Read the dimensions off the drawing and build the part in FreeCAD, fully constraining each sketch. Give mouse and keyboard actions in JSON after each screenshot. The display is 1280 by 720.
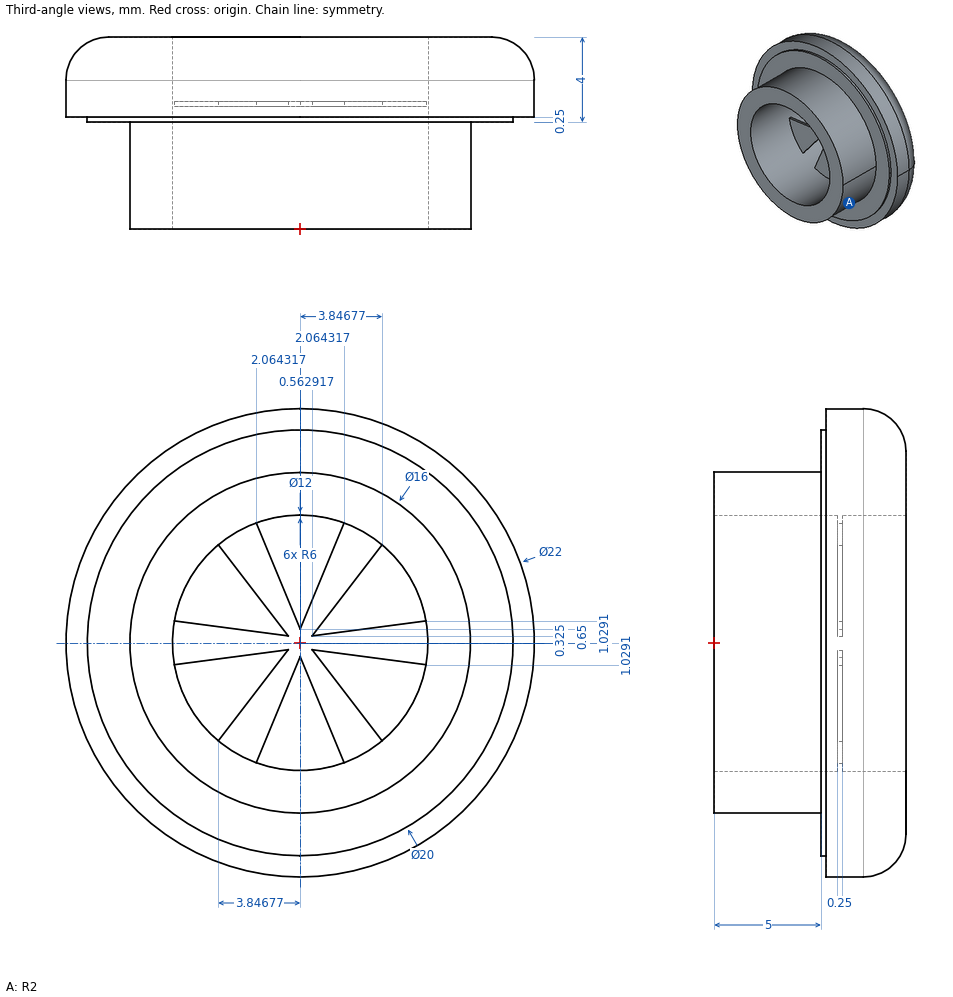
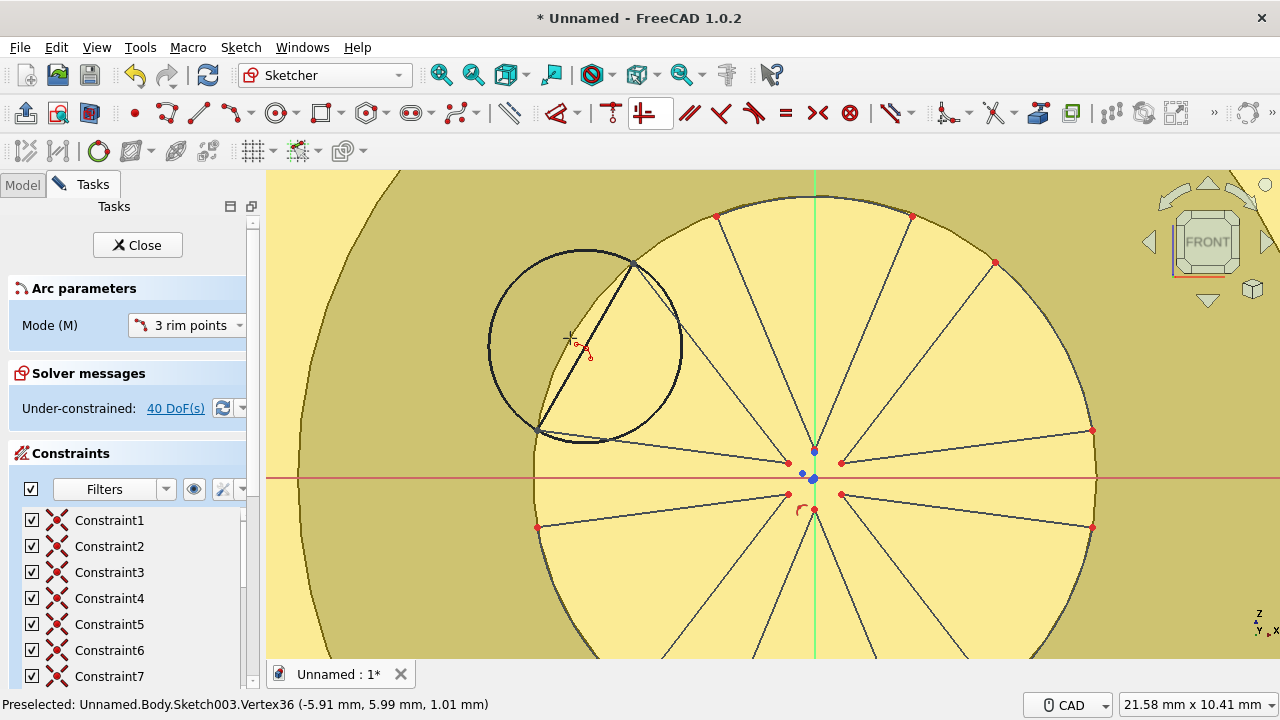
{"action": "left_click", "coordinate": [571, 337]}
{"action": "key", "text": "Escape"}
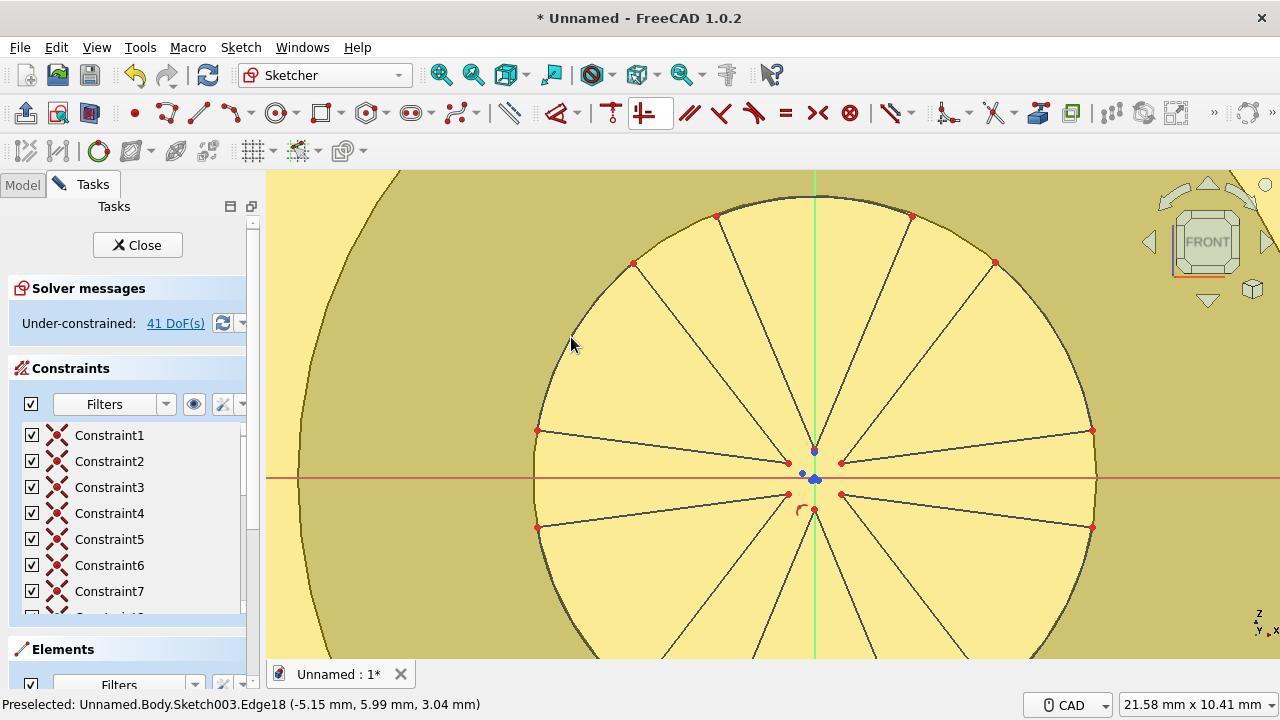
{"action": "left_click", "coordinate": [855, 200]}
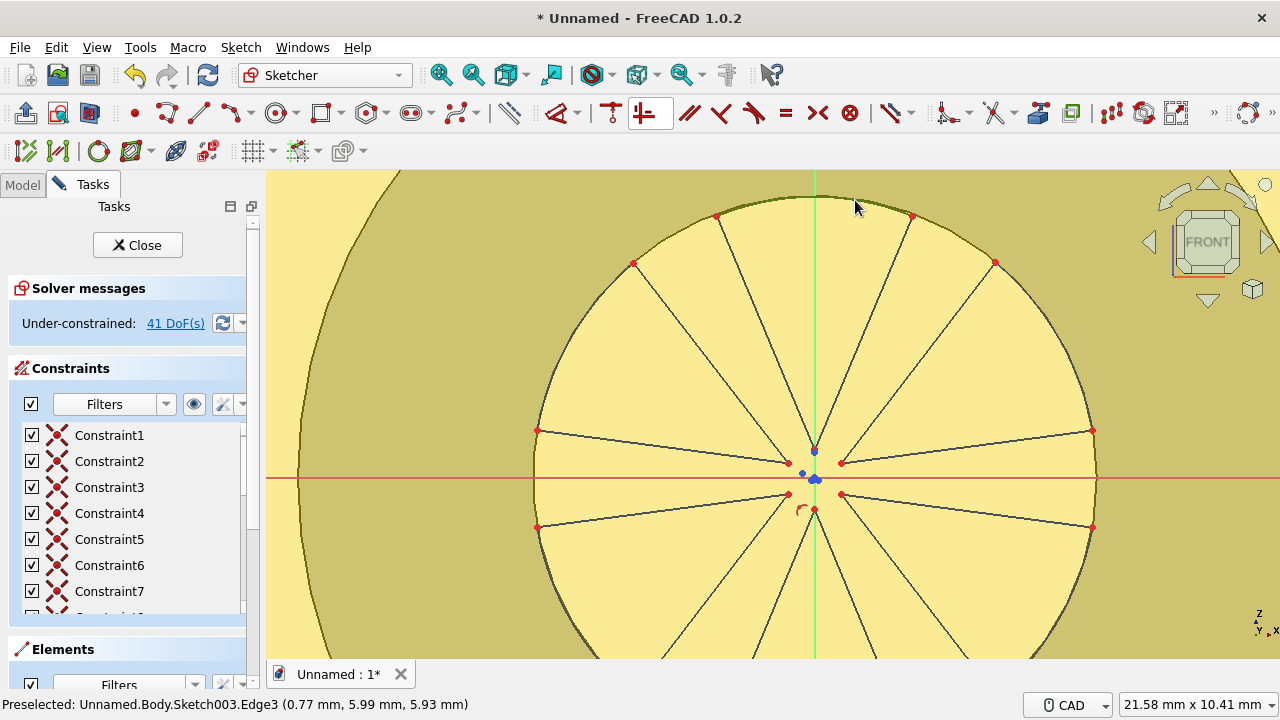
{"action": "left_click", "coordinate": [1076, 374]}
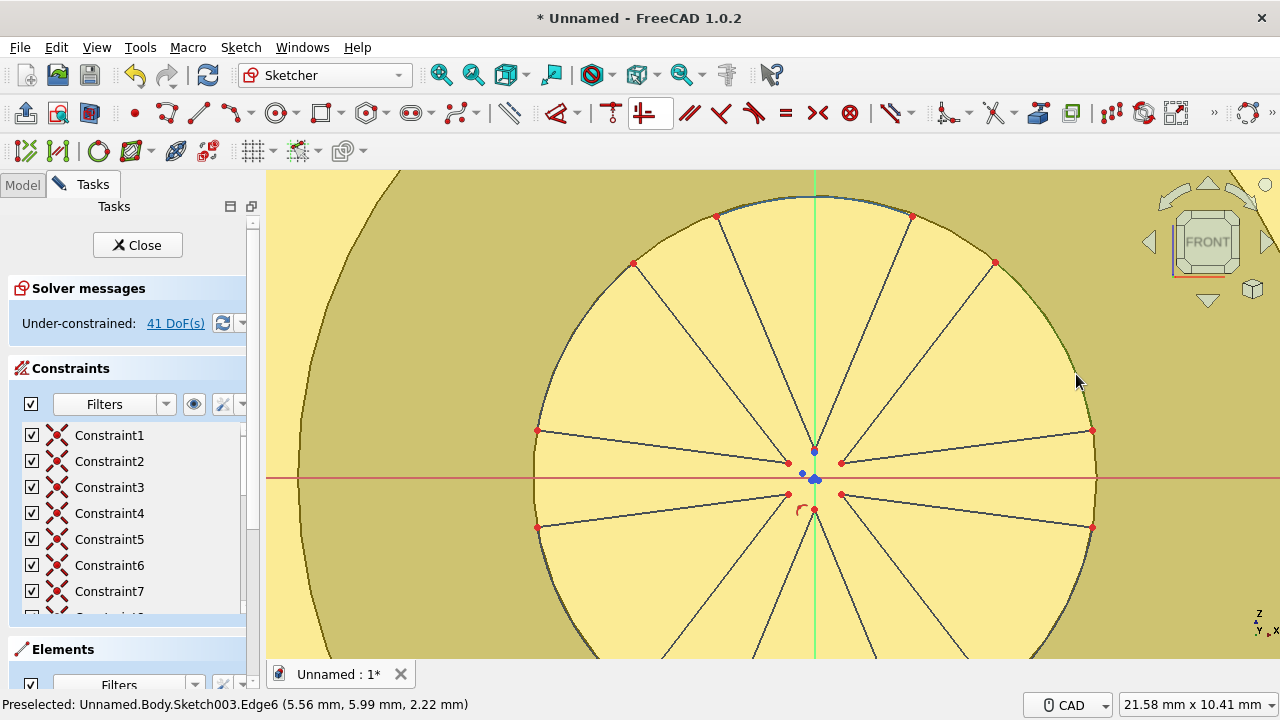
{"action": "key", "text": "c"}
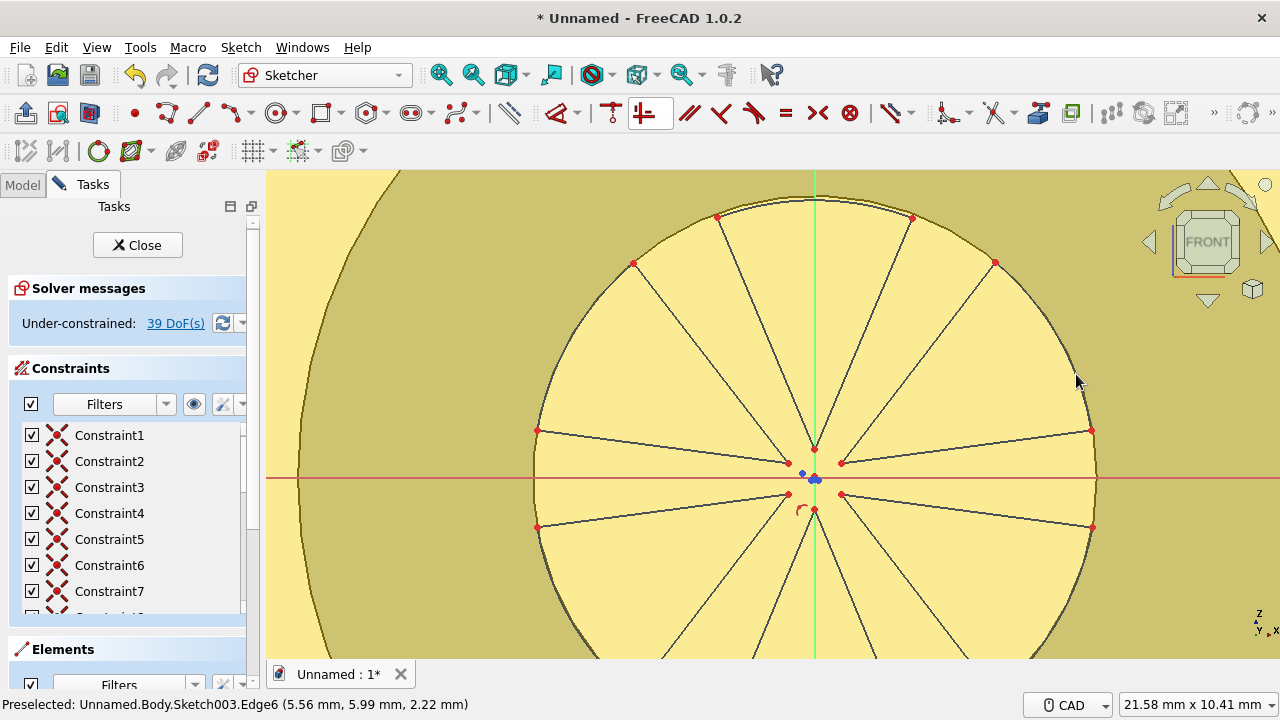
{"action": "left_click", "coordinate": [855, 203]}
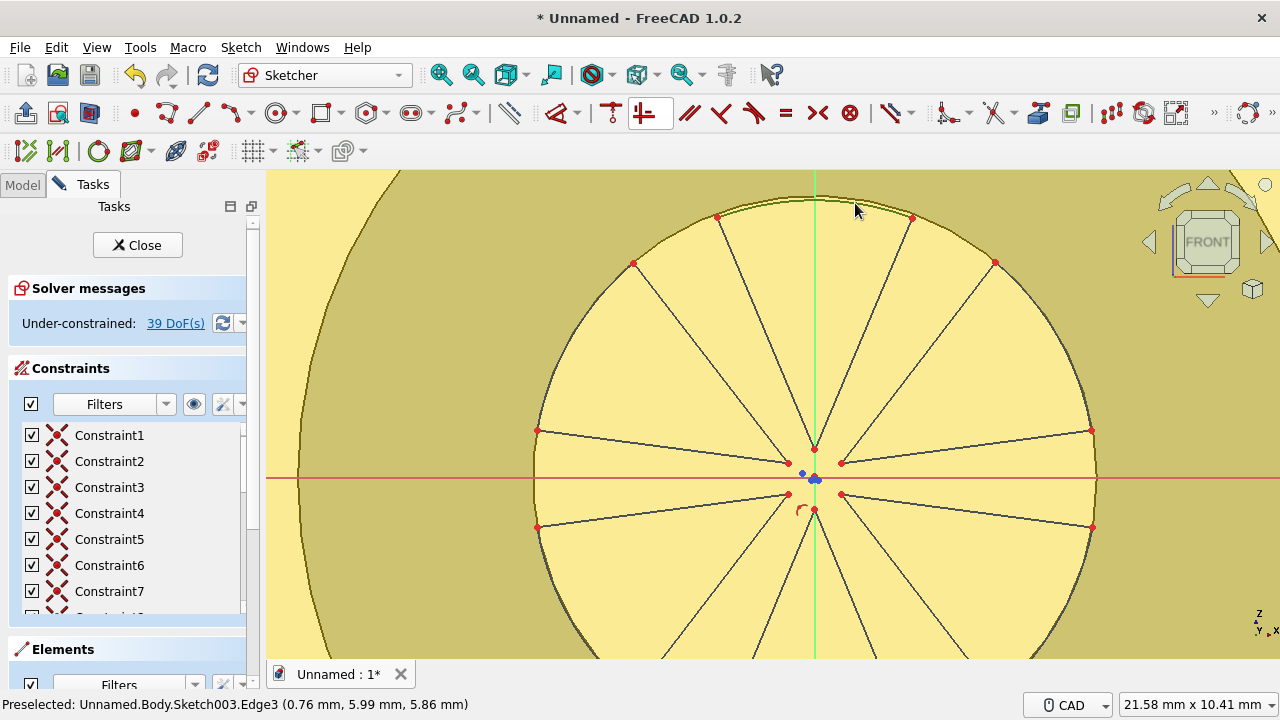
{"action": "left_click", "coordinate": [1076, 584]}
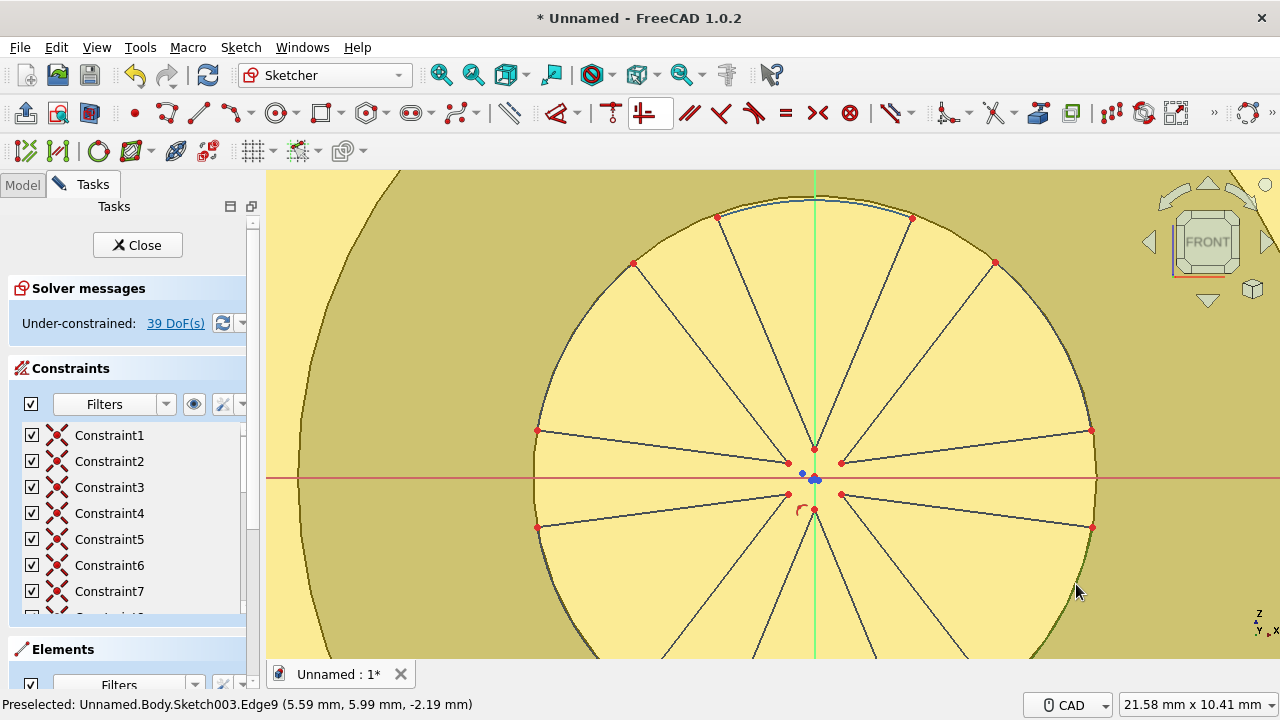
{"action": "left_click", "coordinate": [612, 114]}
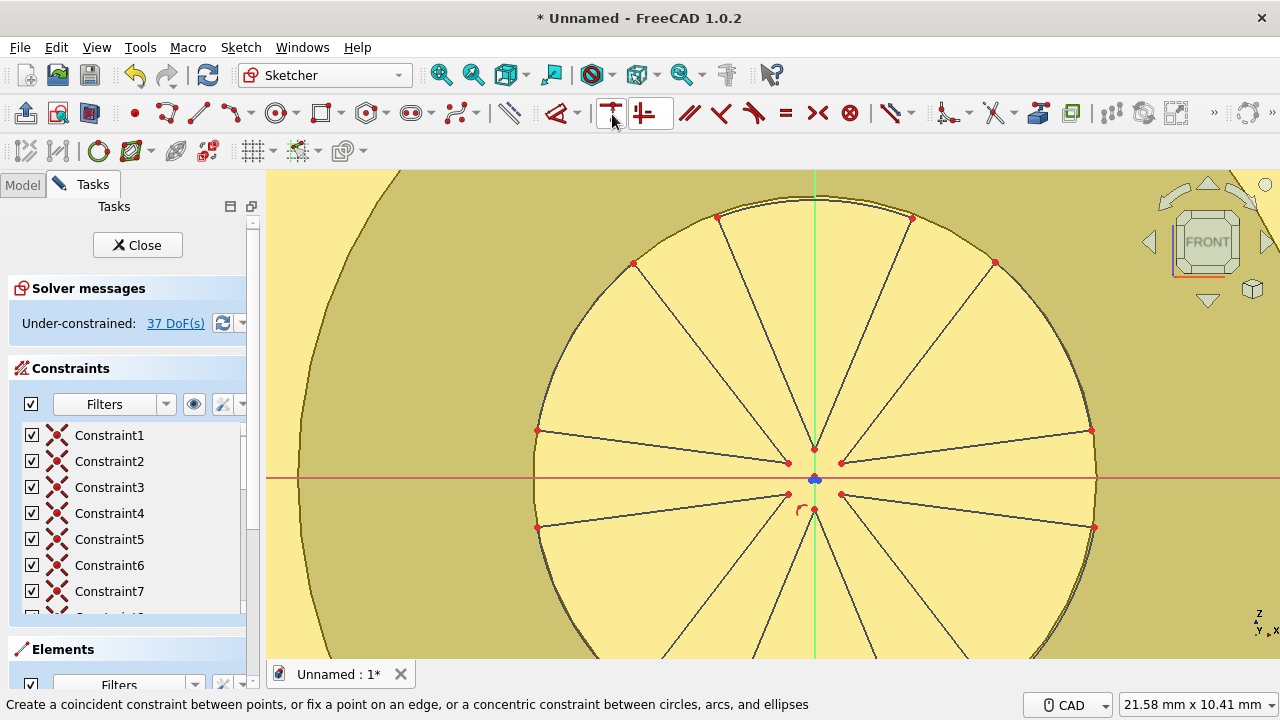
{"action": "left_click", "coordinate": [855, 203]}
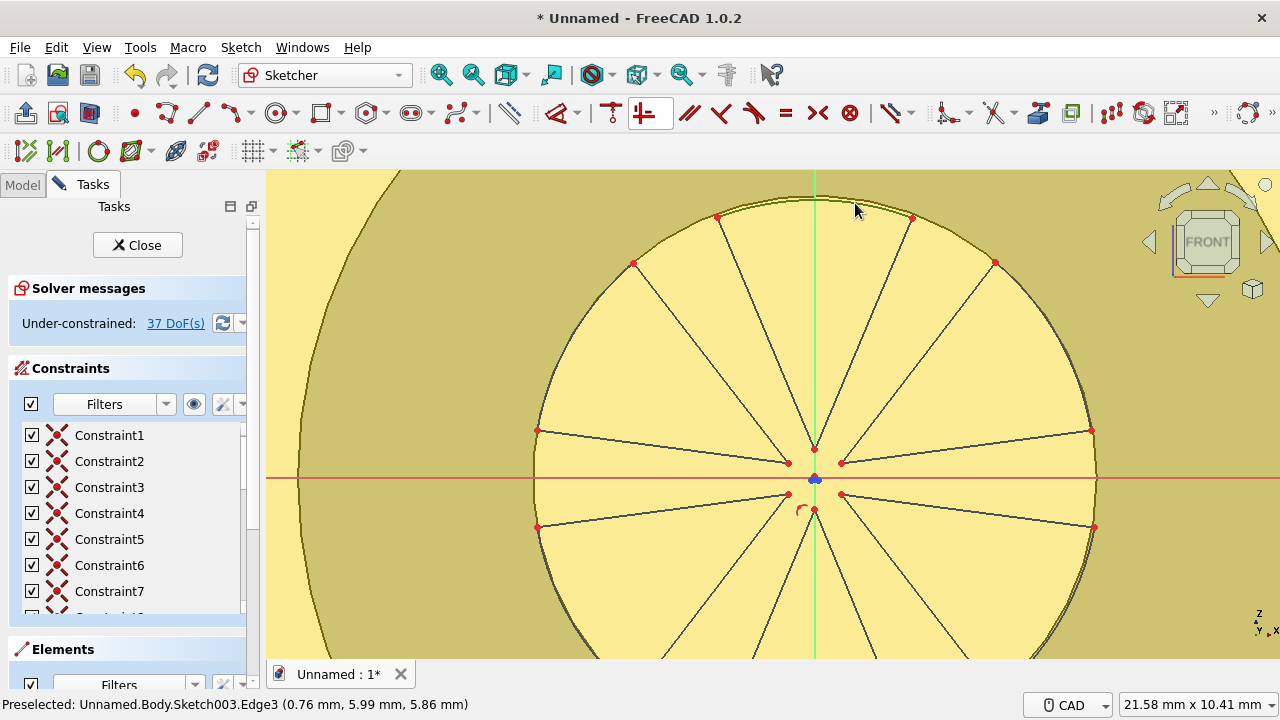
{"action": "scroll", "coordinate": [570, 338], "scroll_direction": "down", "scroll_amount": 3}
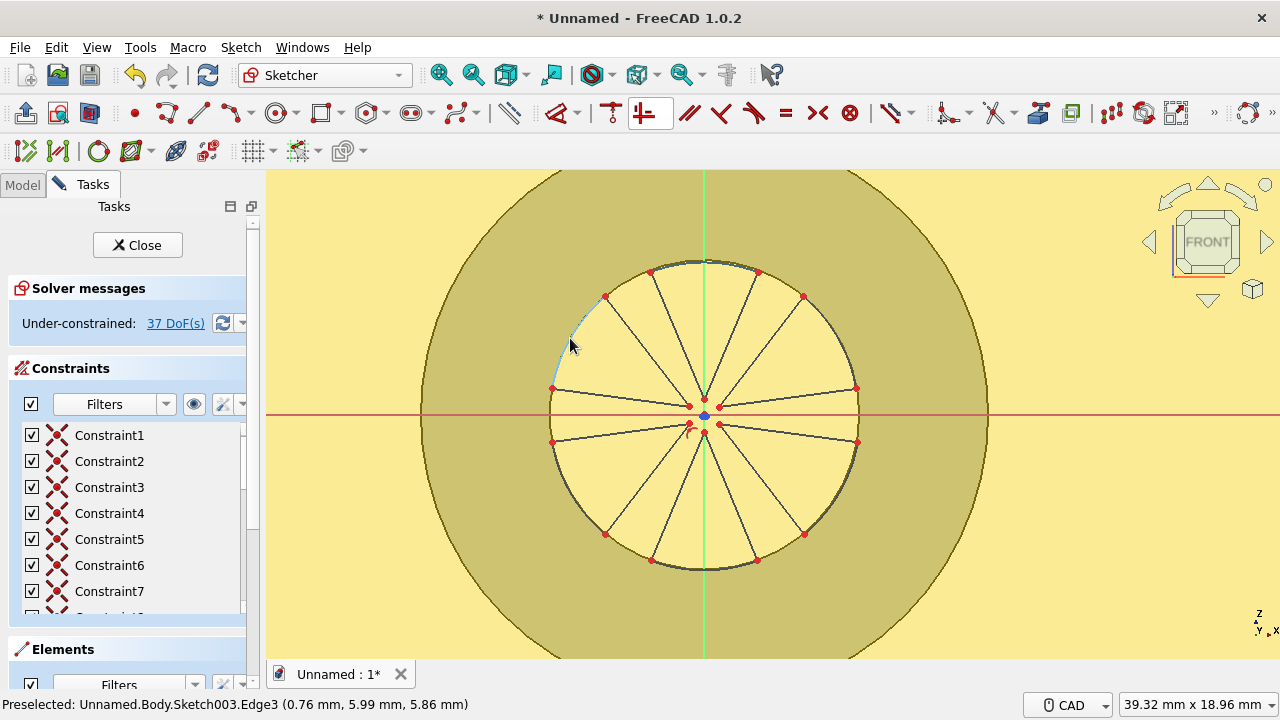
{"action": "left_click", "coordinate": [683, 569]}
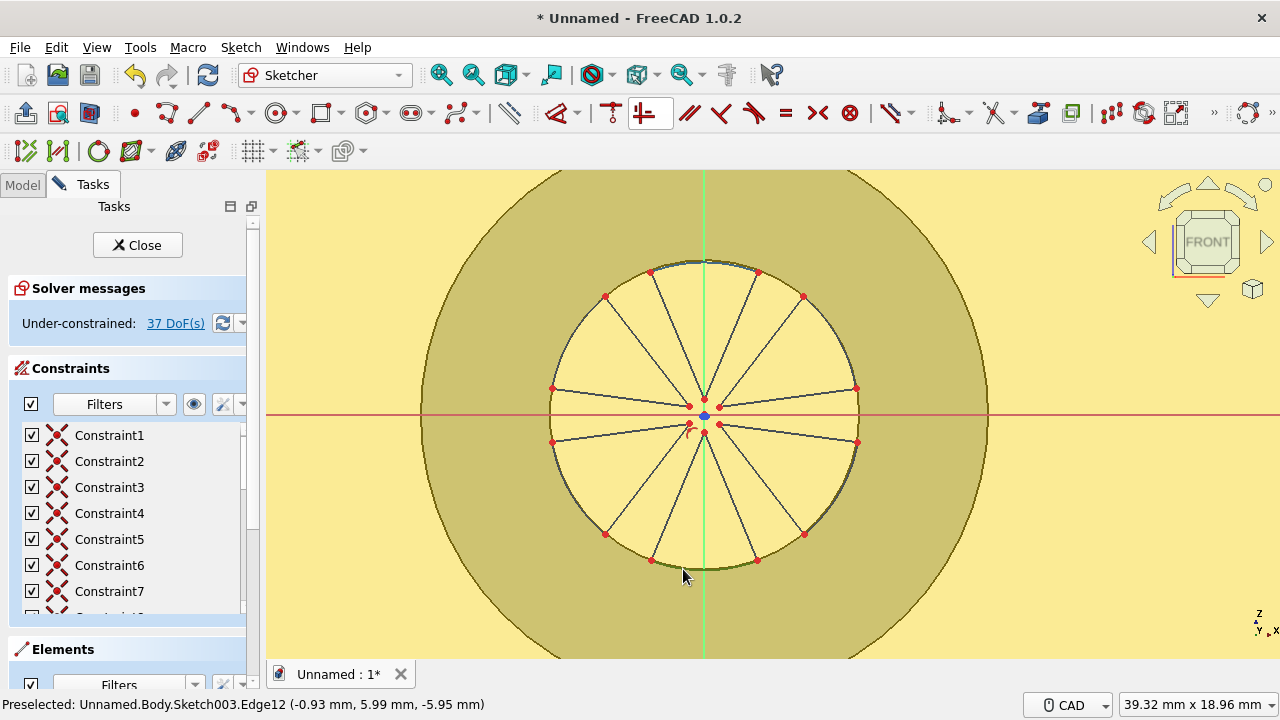
{"action": "key", "text": "c"}